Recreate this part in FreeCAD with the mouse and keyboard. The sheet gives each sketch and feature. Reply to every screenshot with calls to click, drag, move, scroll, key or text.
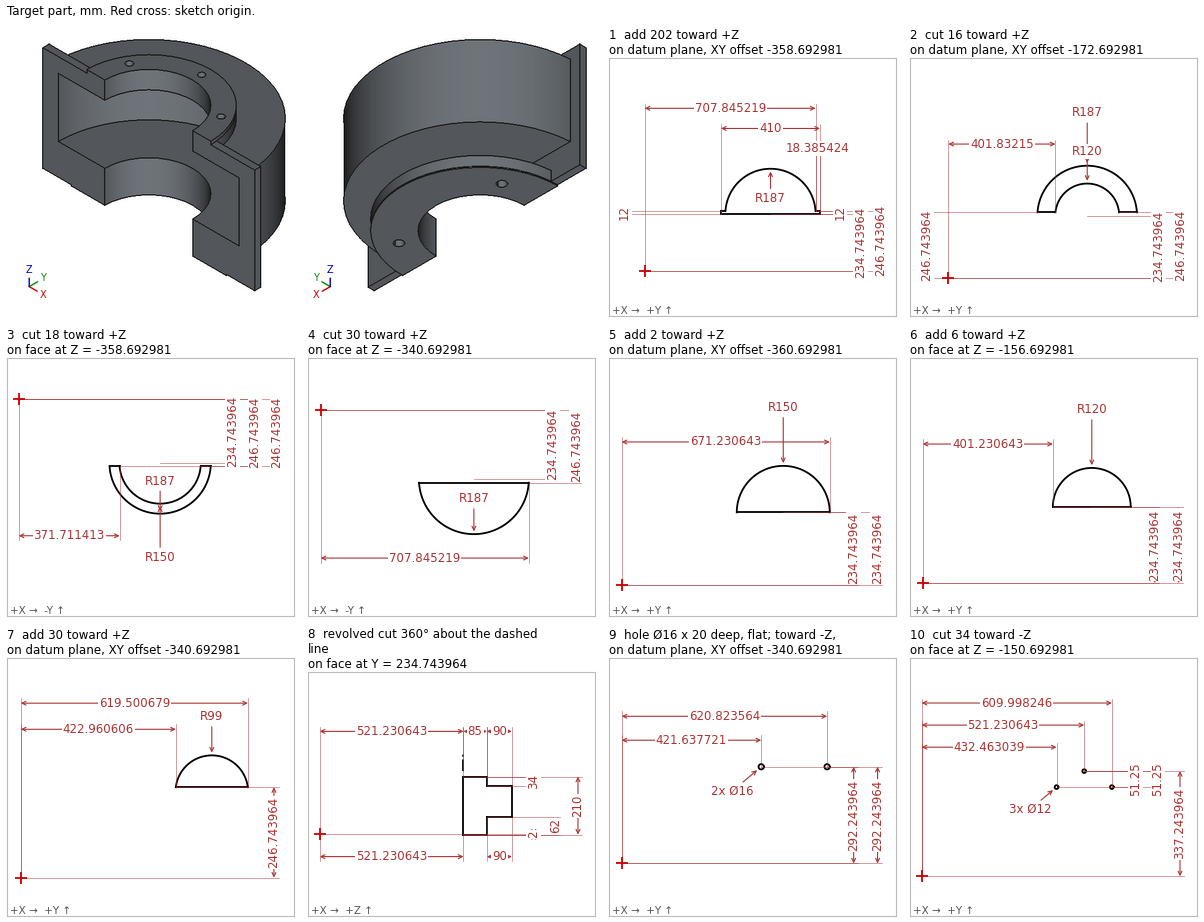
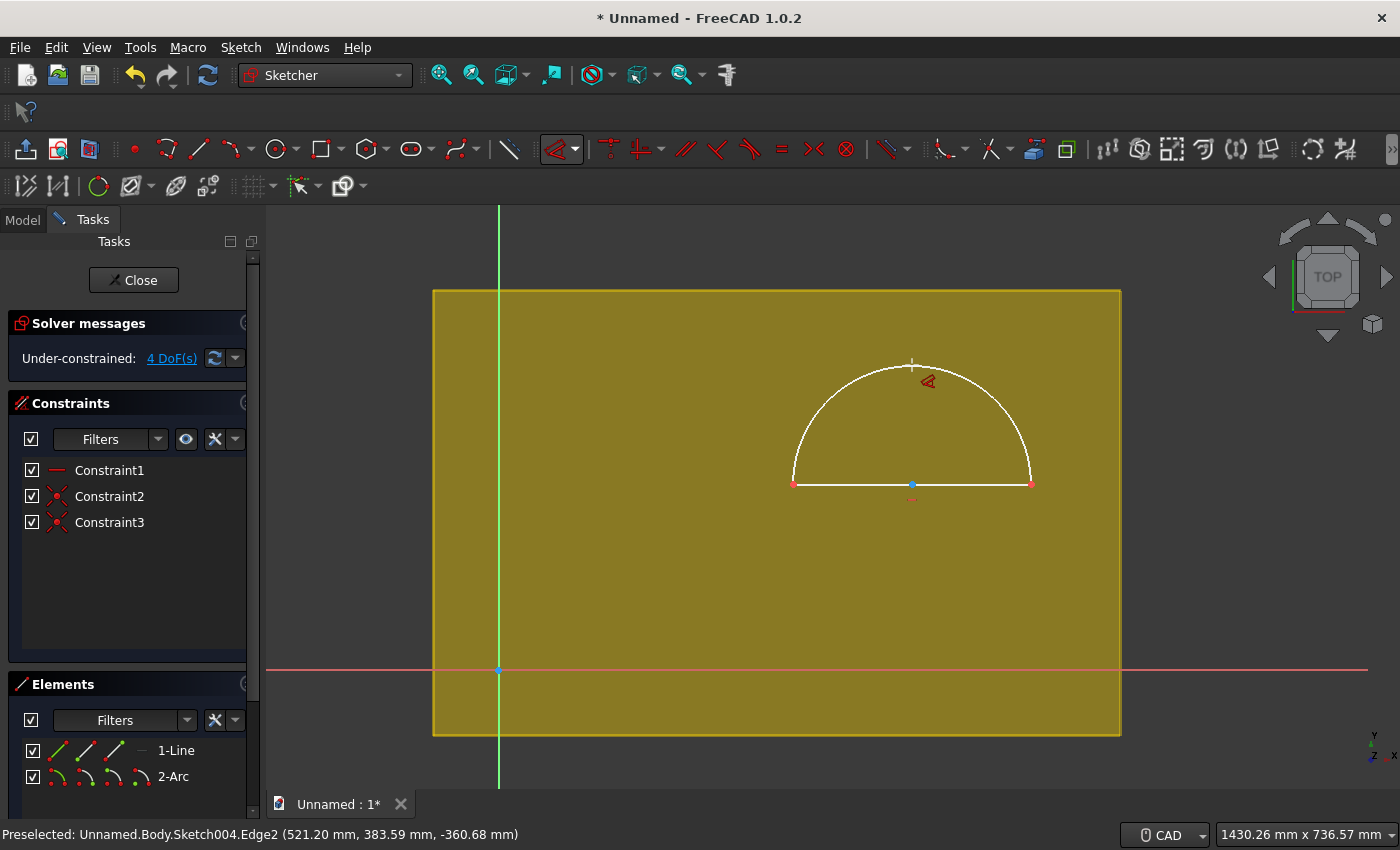
click(982, 389)
click(1001, 363)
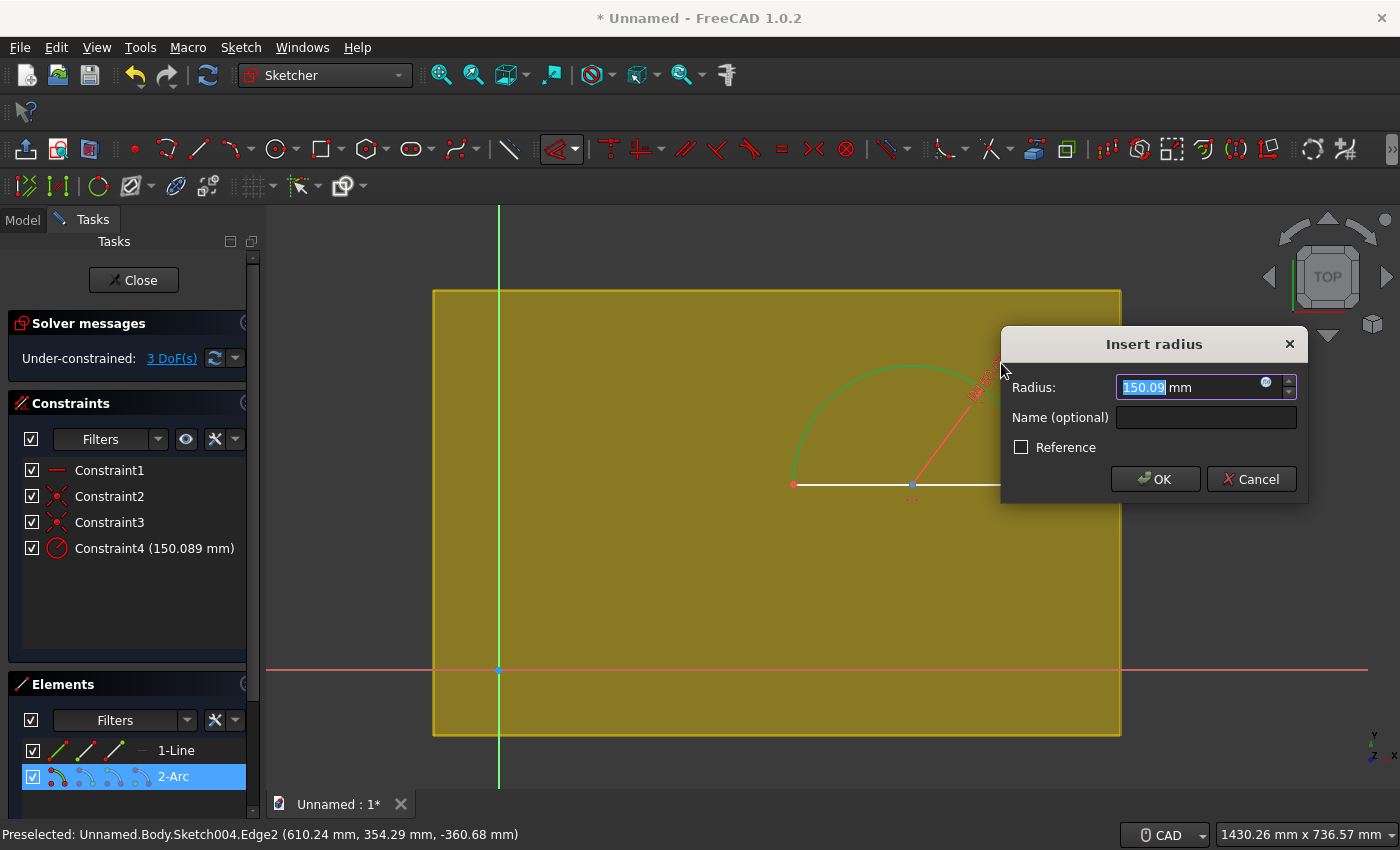
text(150)
key(Return)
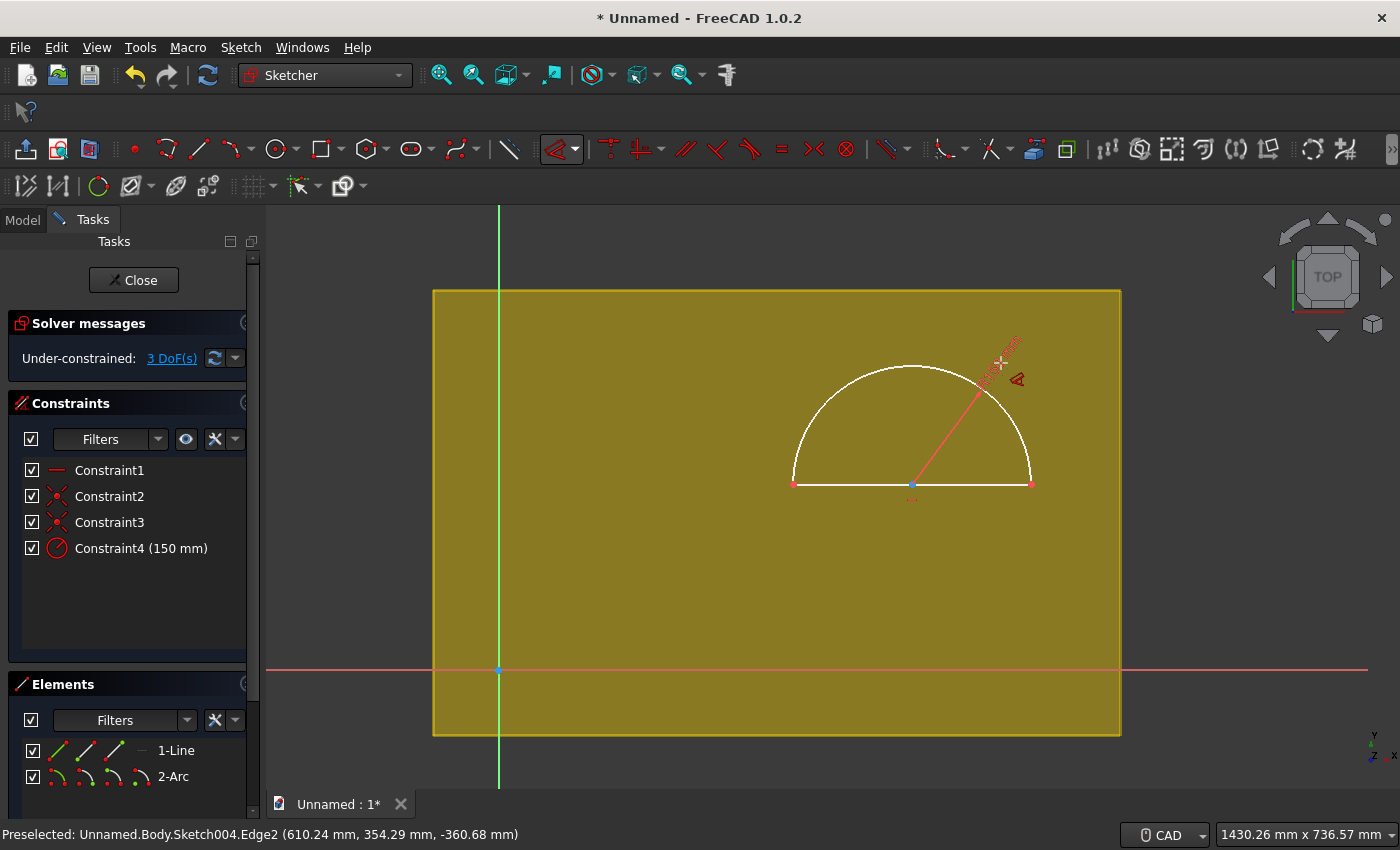
click(1031, 485)
click(765, 704)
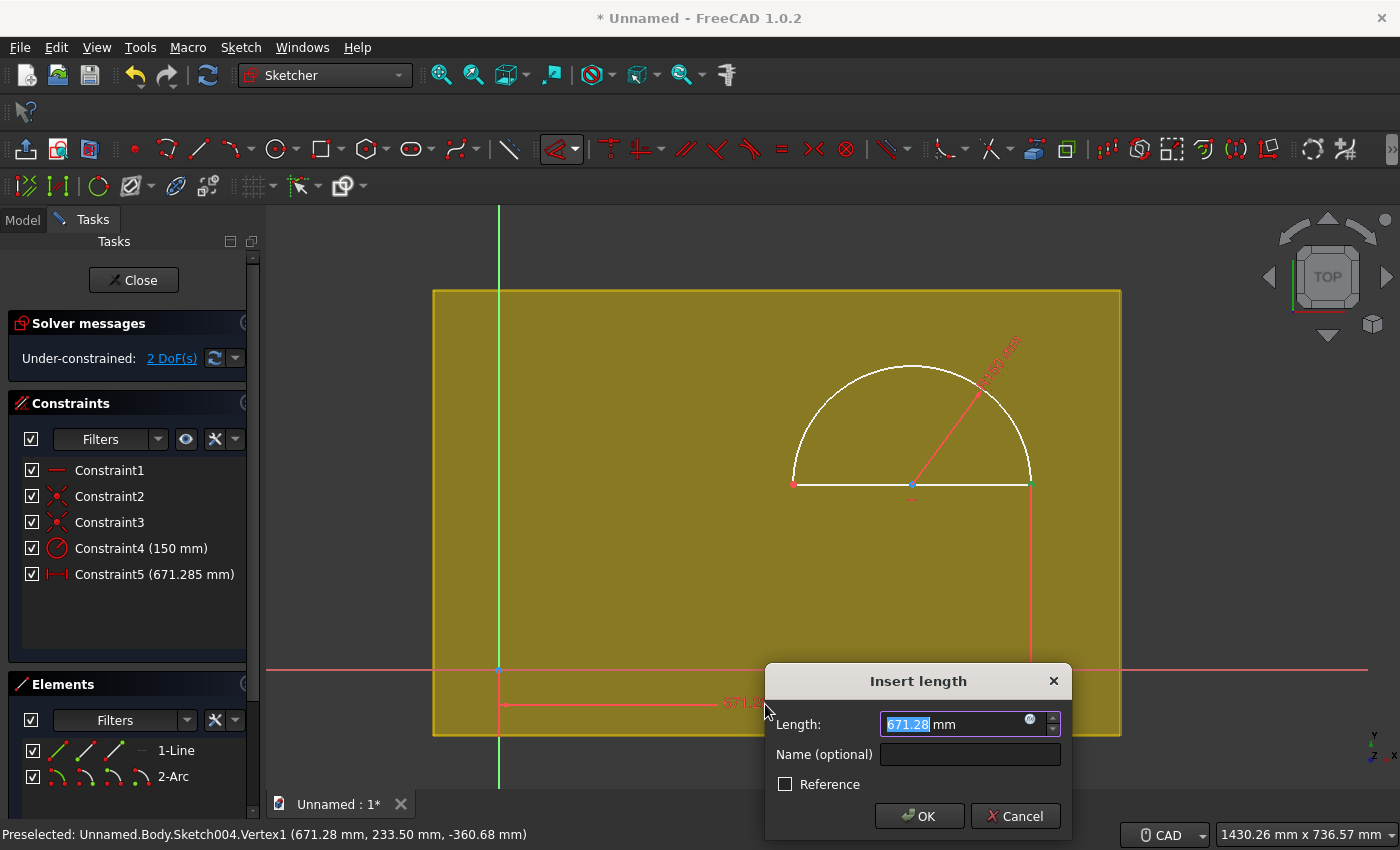
text(671.230643)
key(Return)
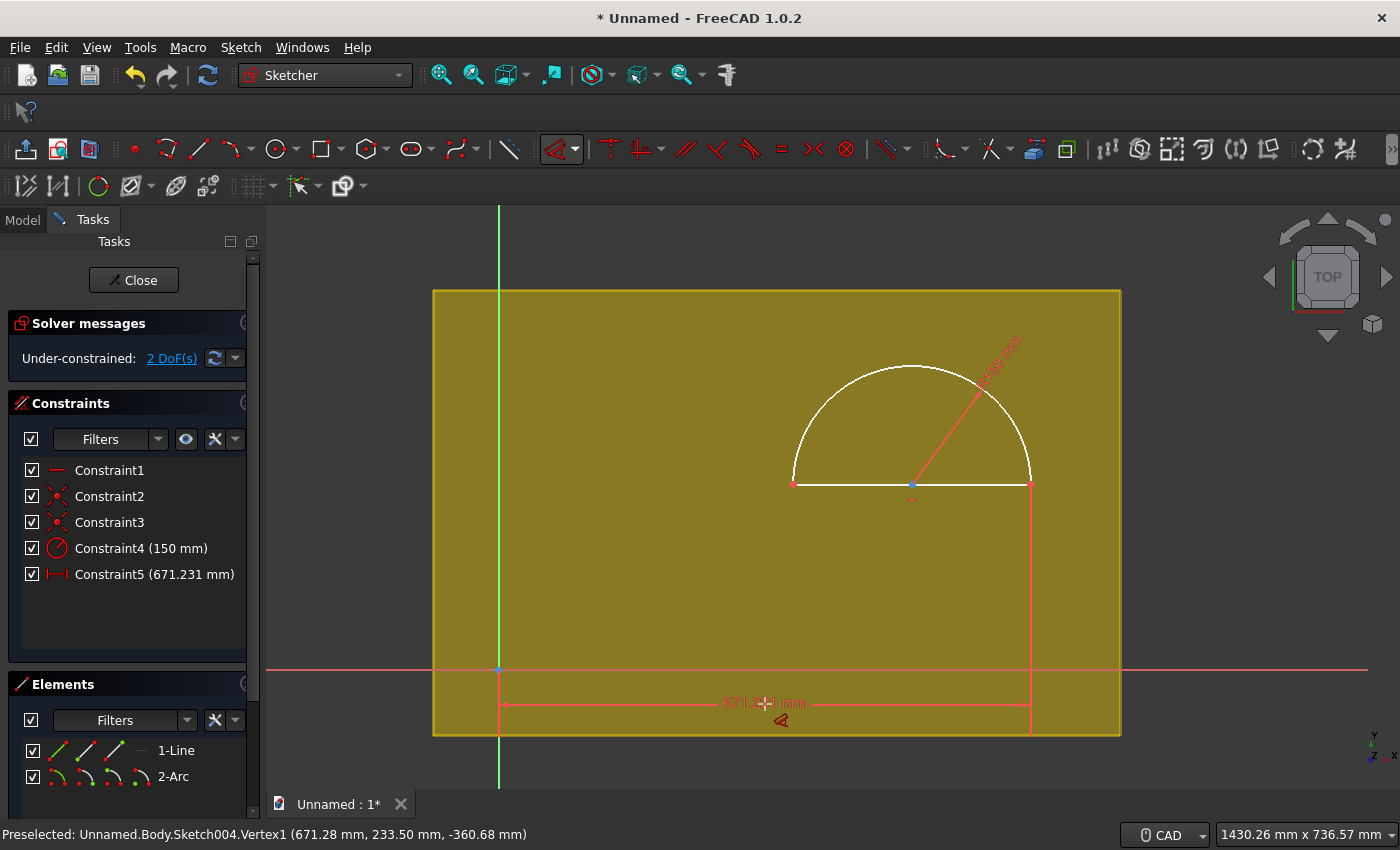
click(1031, 485)
click(1065, 578)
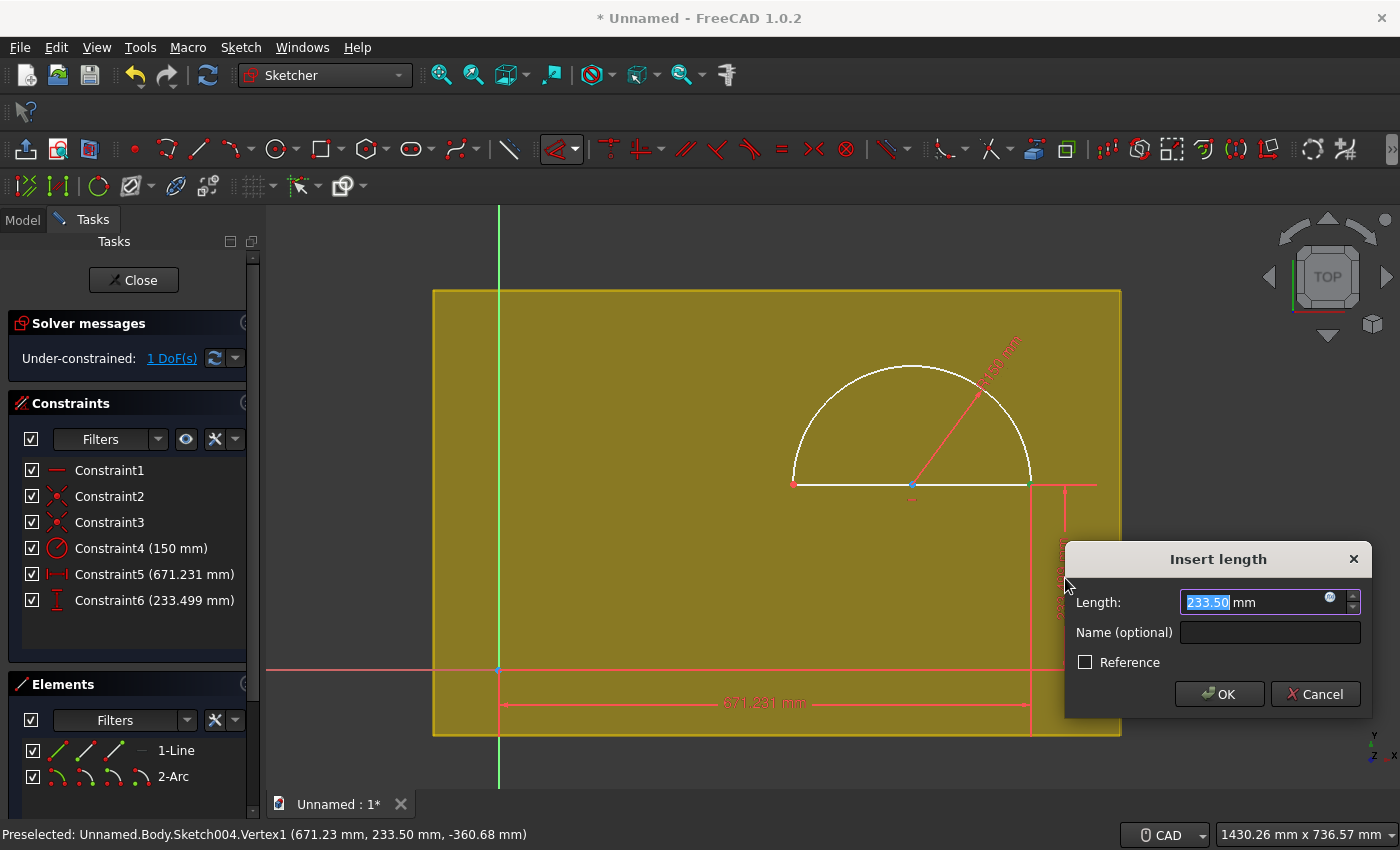
text(234.743964)
key(Return)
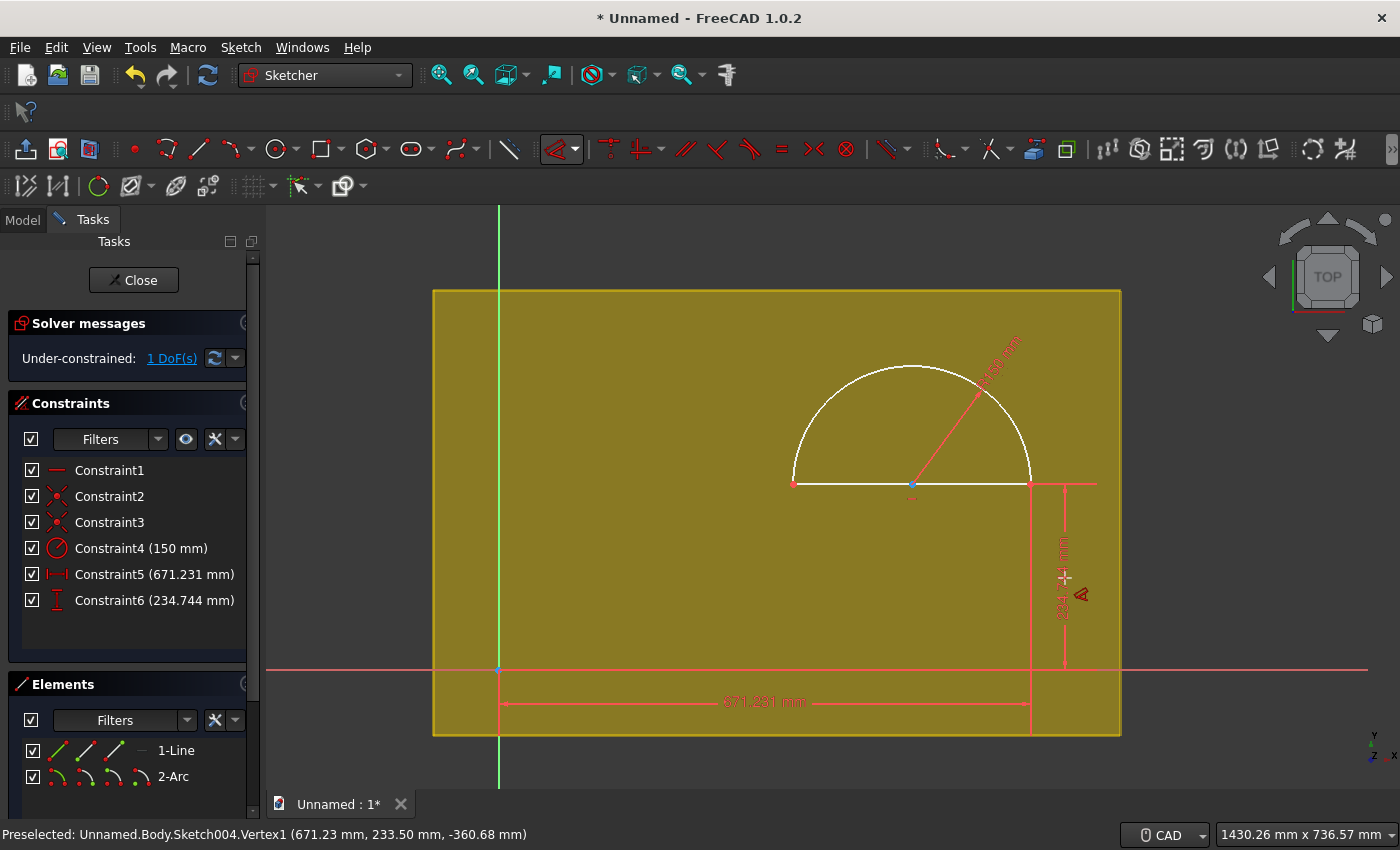
click(912, 485)
click(465, 578)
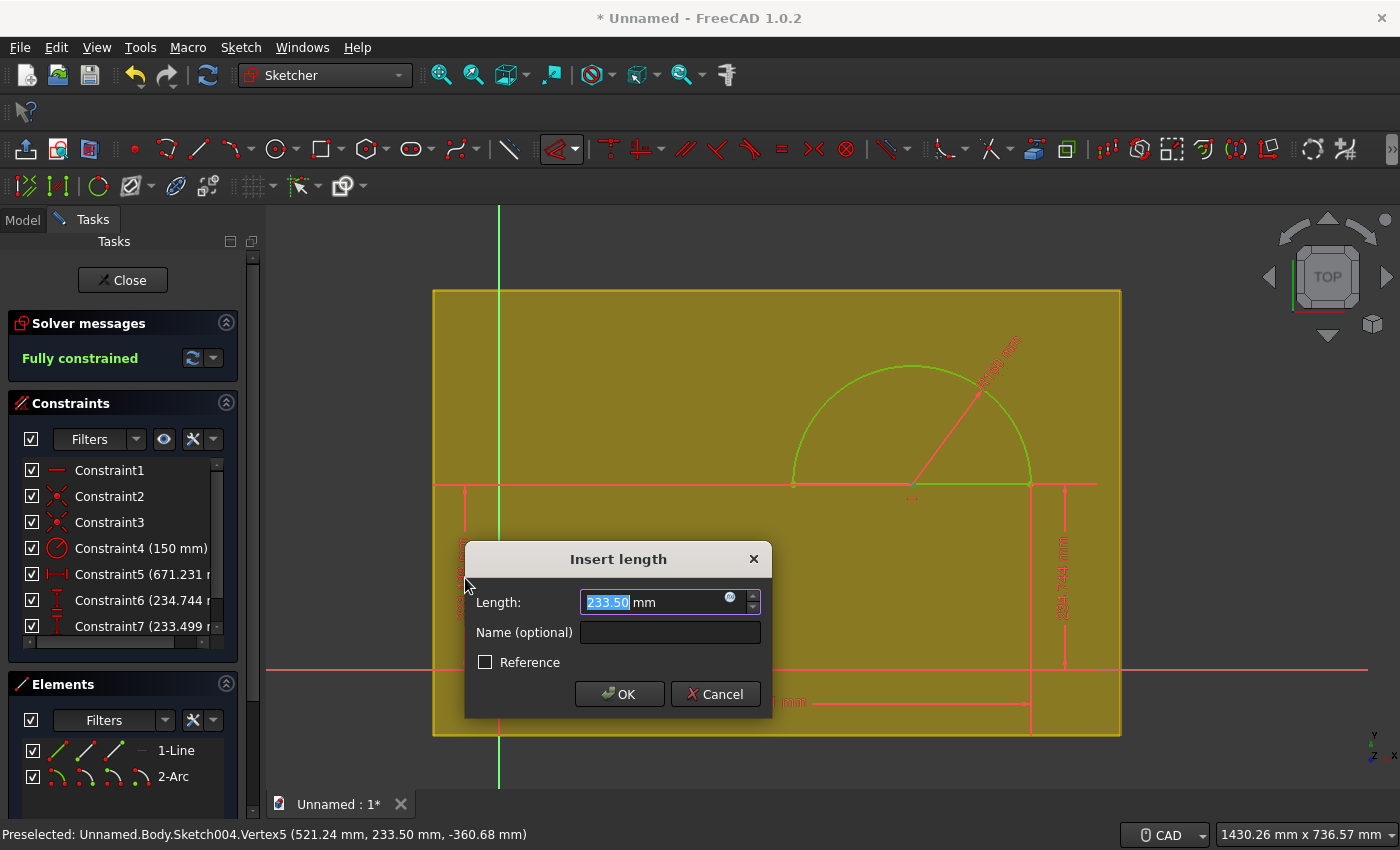
text(234.743964)
key(Return)
key(Escape)